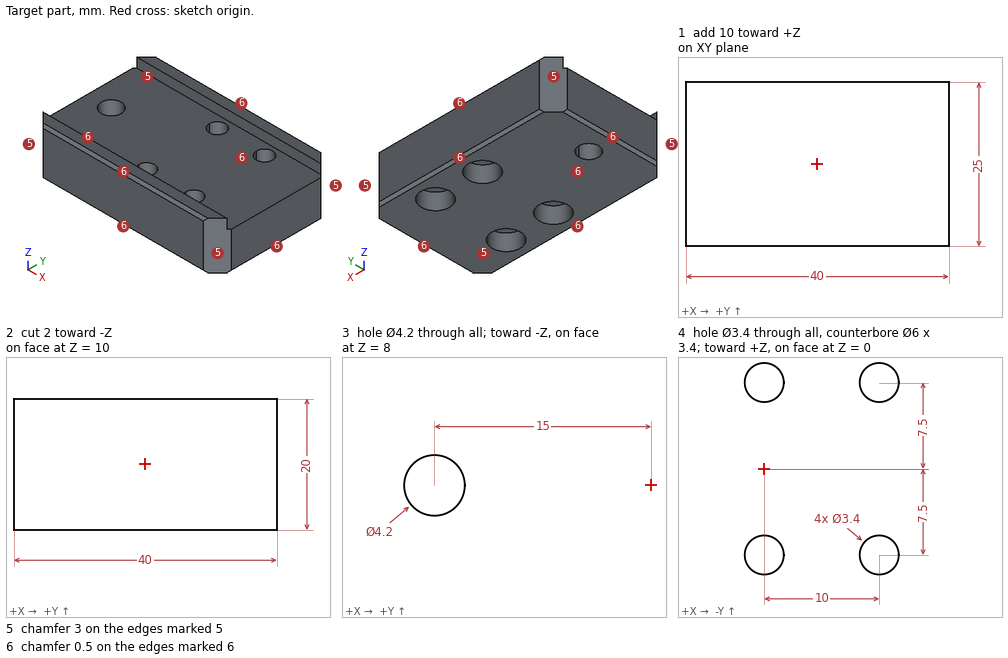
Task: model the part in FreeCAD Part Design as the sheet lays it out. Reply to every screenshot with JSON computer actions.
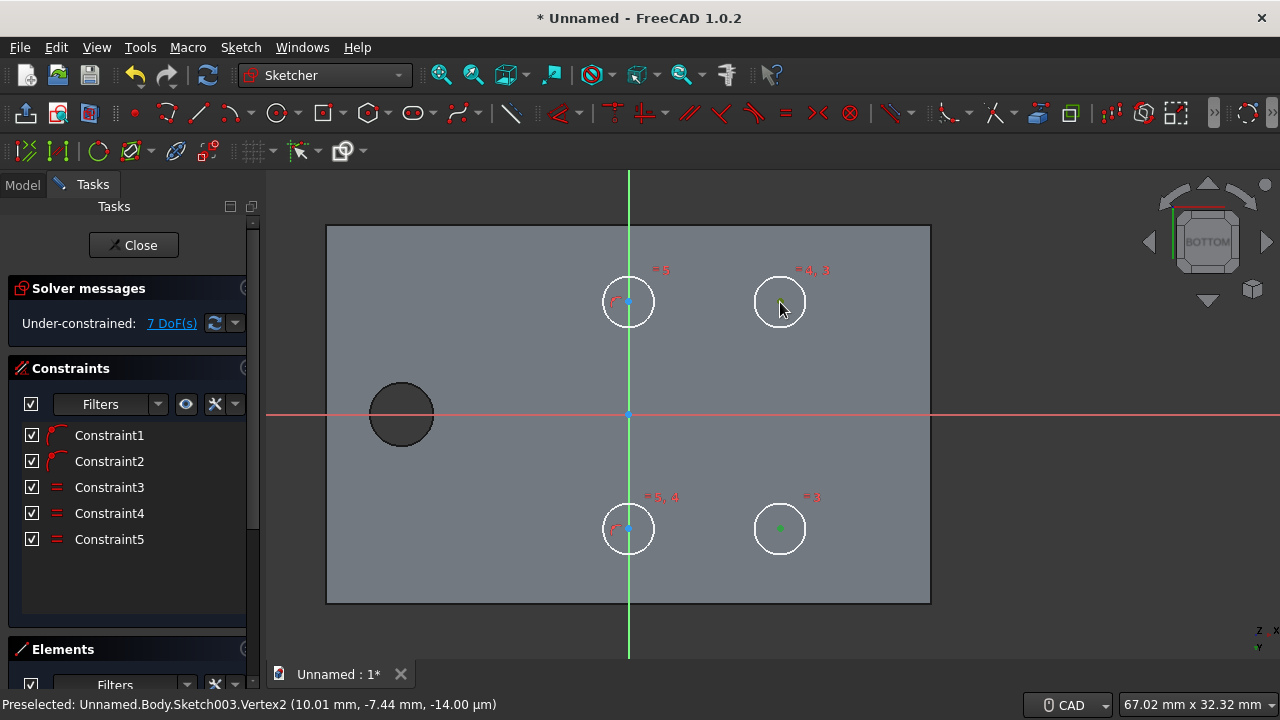
{"action": "key", "text": "v"}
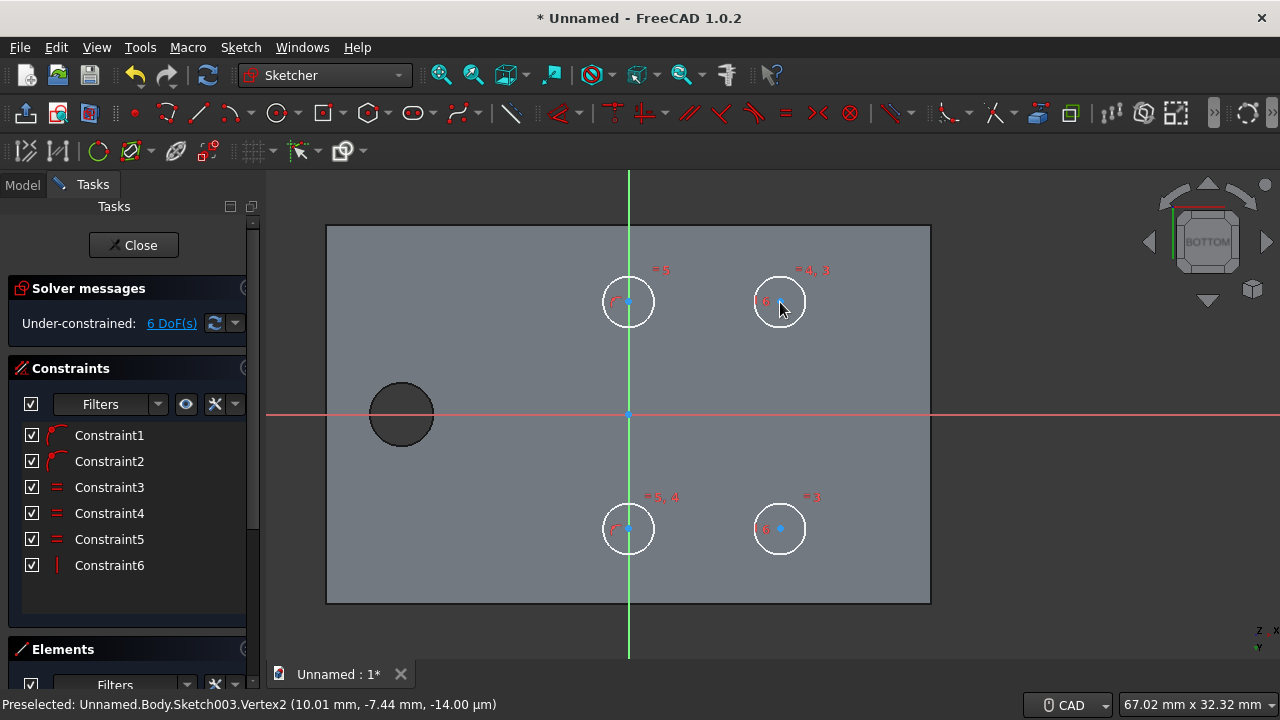
{"action": "left_click", "coordinate": [780, 529]}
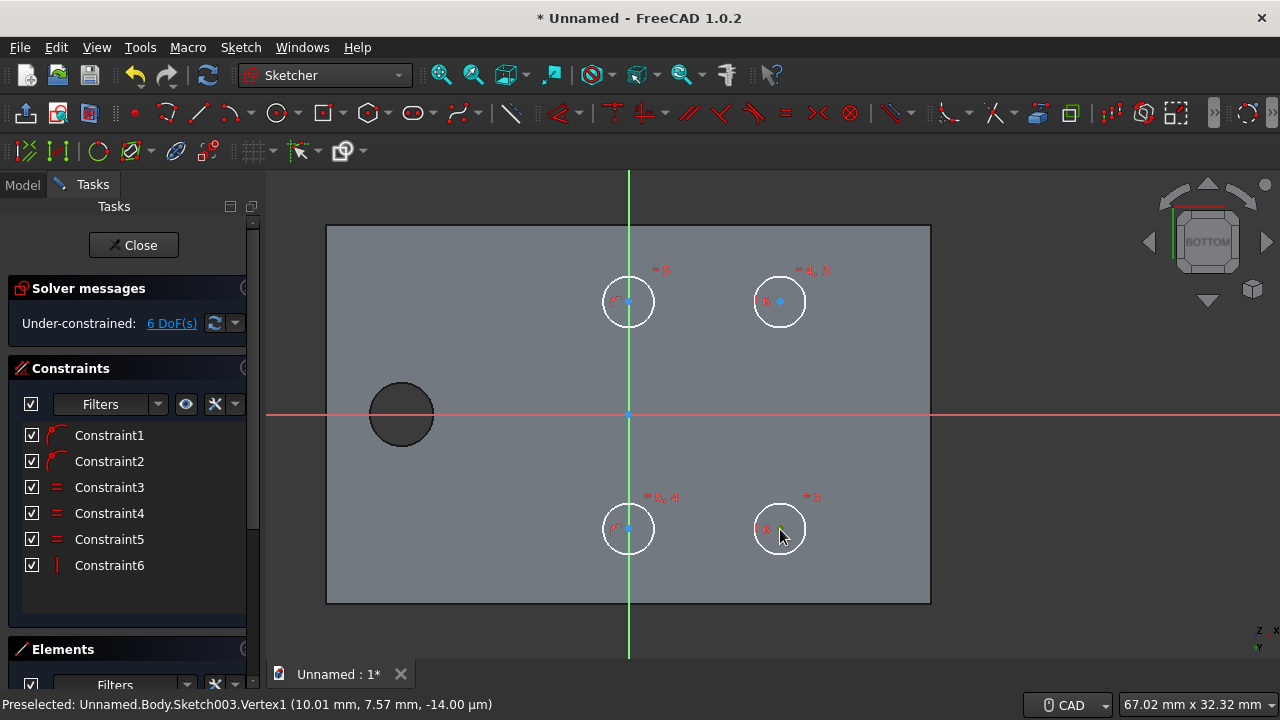
{"action": "left_click", "coordinate": [629, 529]}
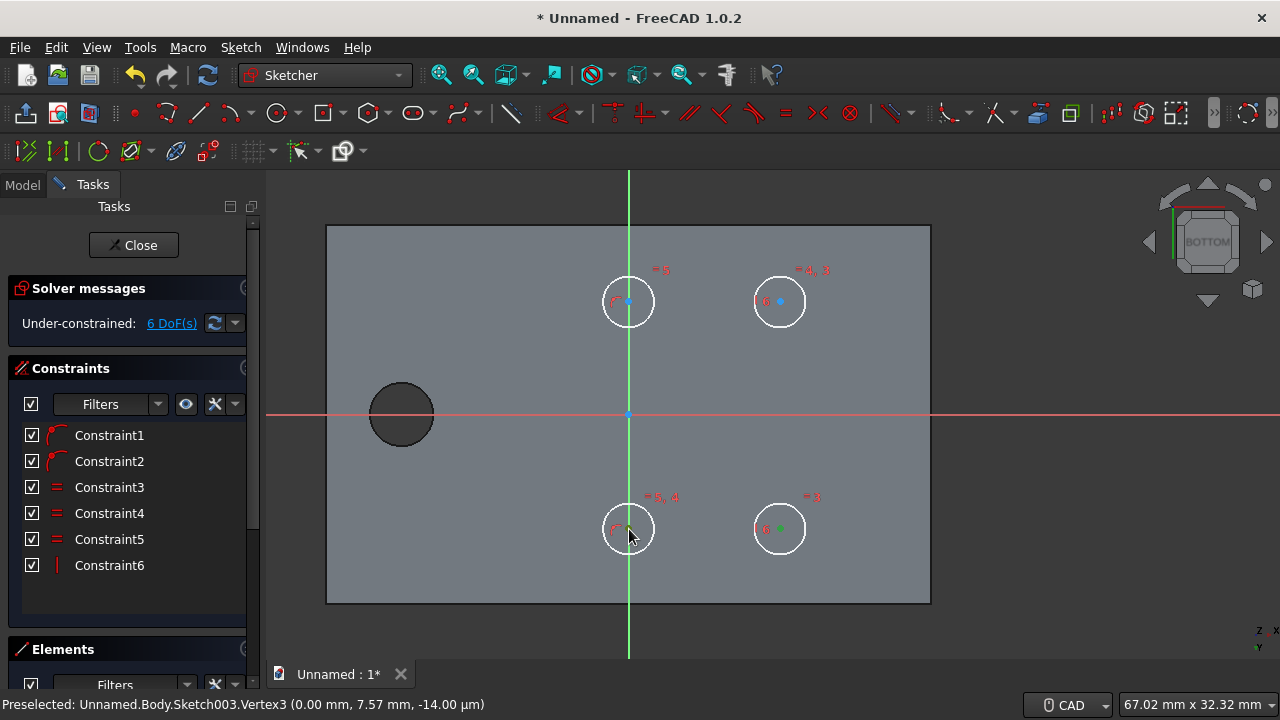
{"action": "key", "text": "h"}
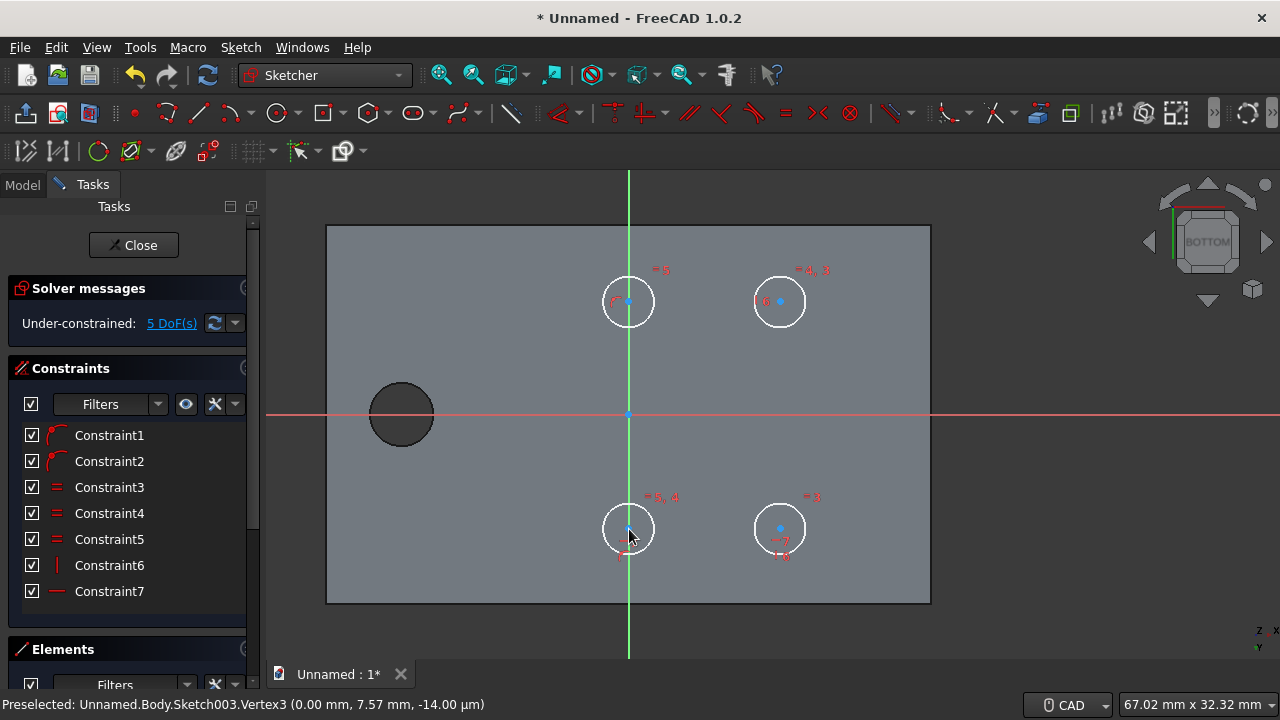
{"action": "left_click", "coordinate": [780, 302]}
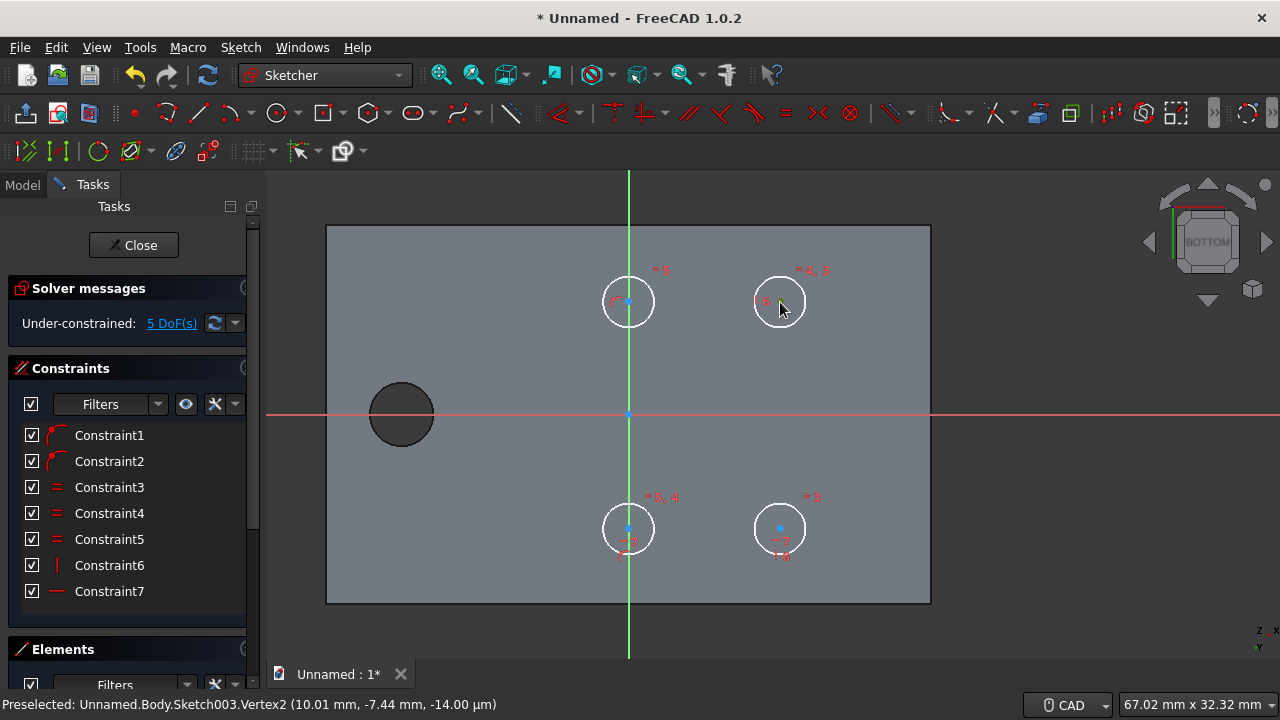
{"action": "left_click", "coordinate": [629, 302]}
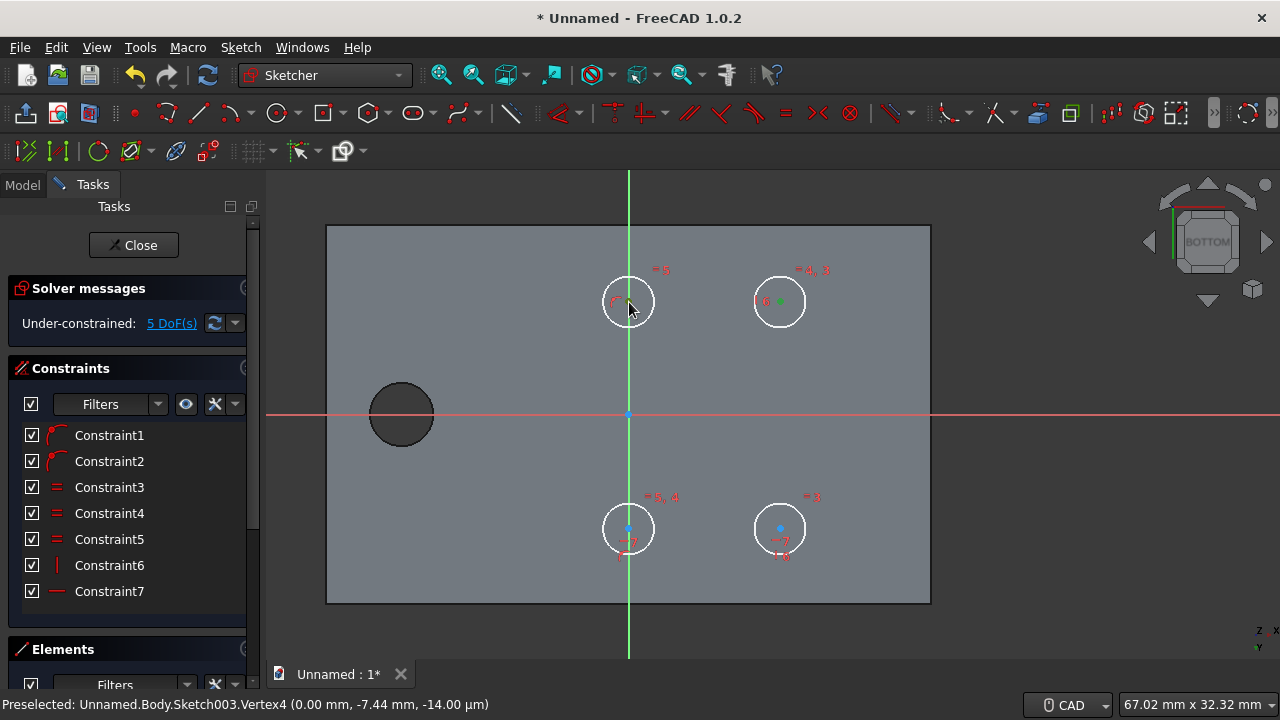
{"action": "left_click", "coordinate": [668, 114]}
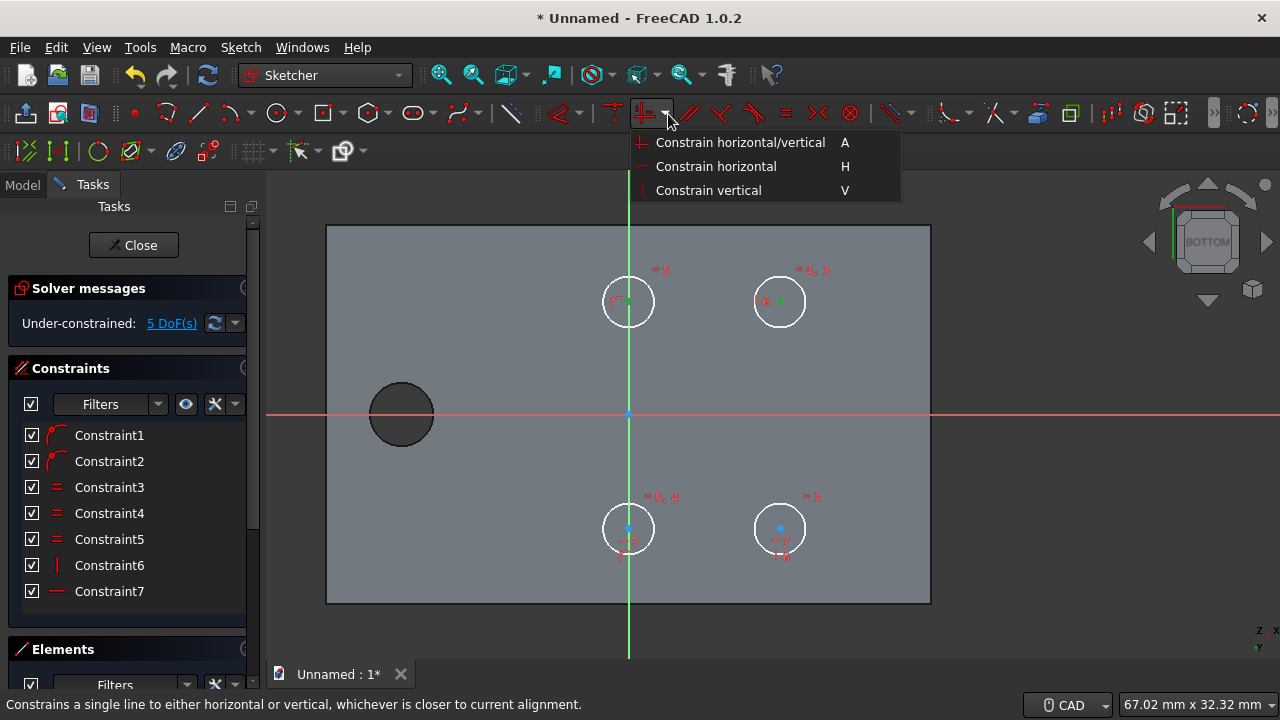
{"action": "left_click", "coordinate": [766, 166]}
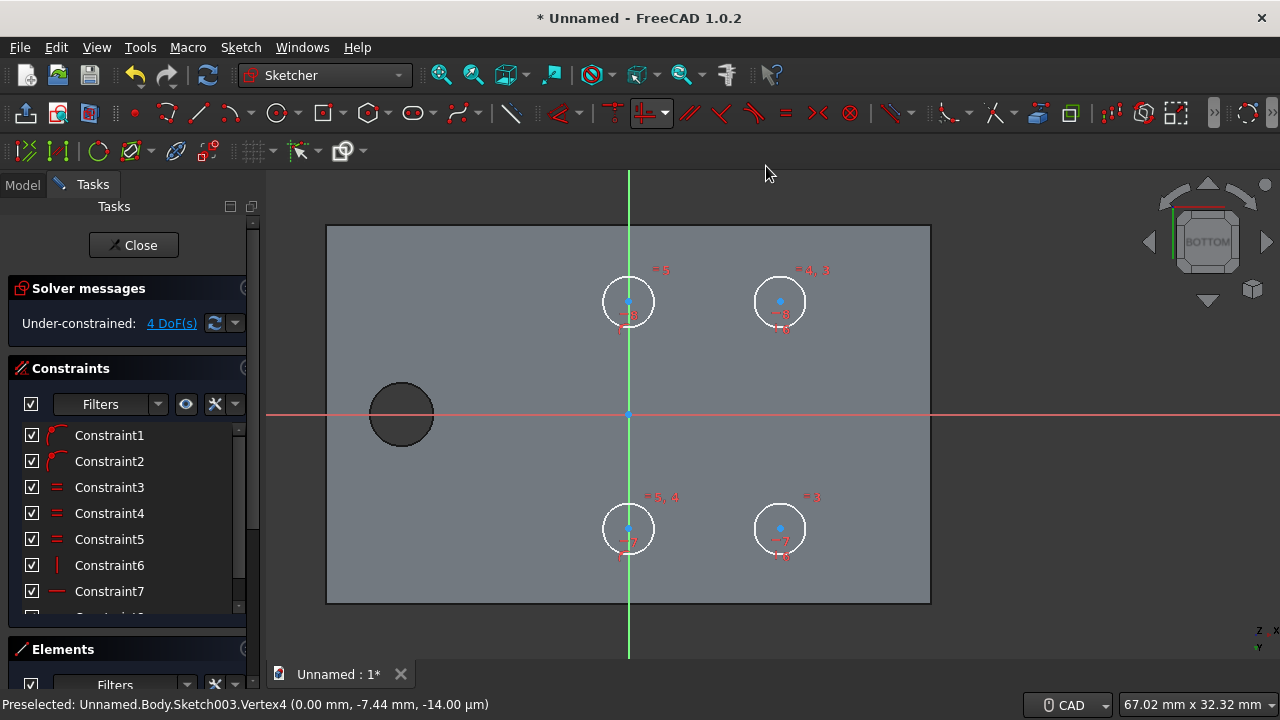
{"action": "left_click", "coordinate": [558, 114]}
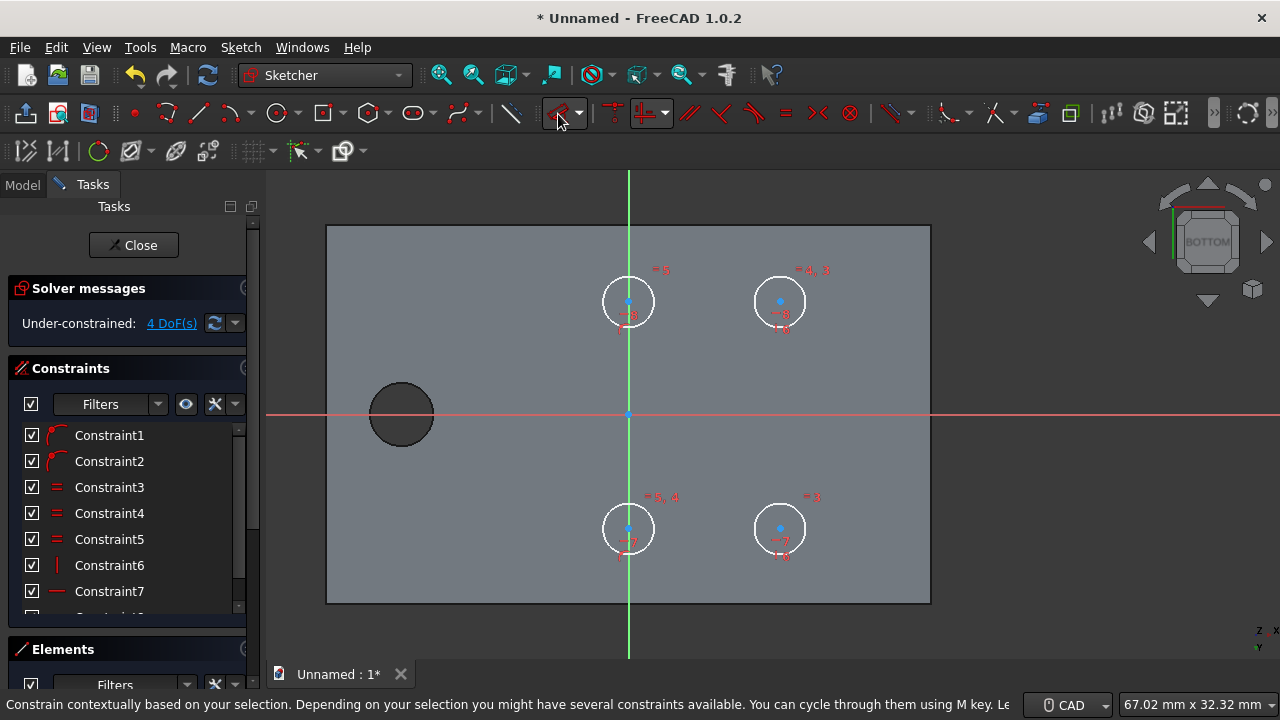
{"action": "left_click", "coordinate": [798, 511]}
{"action": "left_click", "coordinate": [821, 488]}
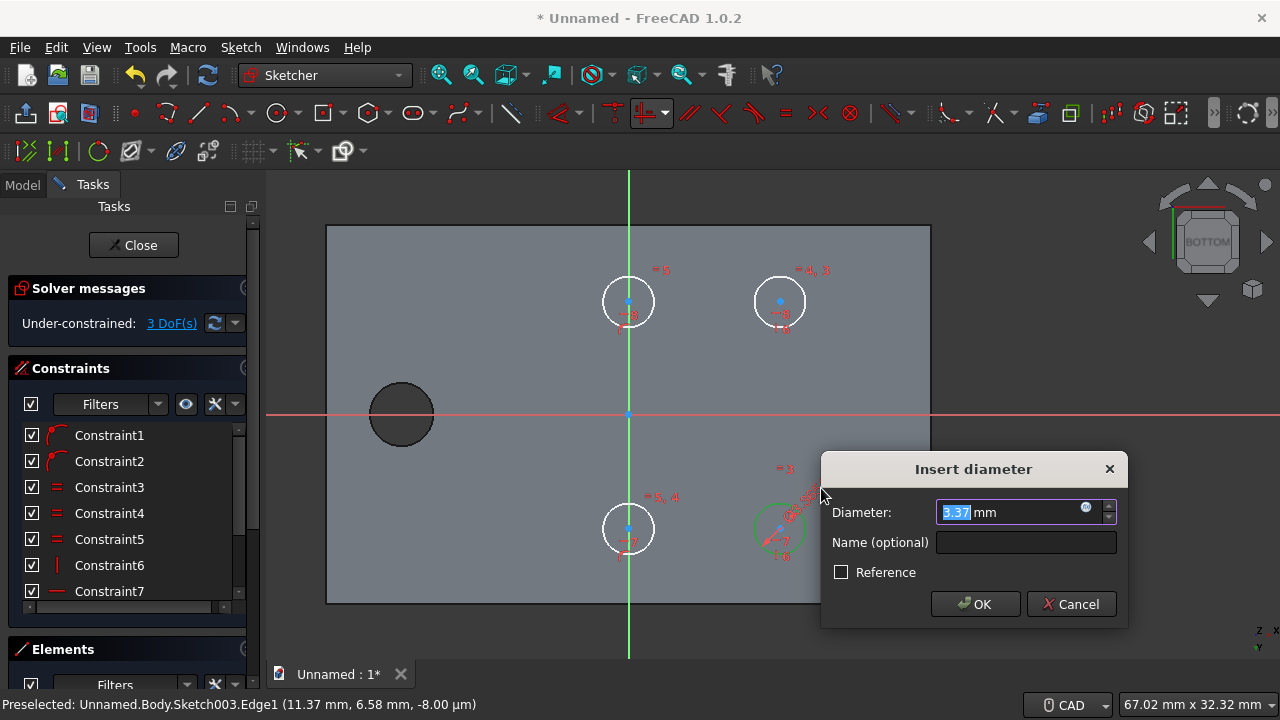
{"action": "type", "text": "3.4"}
{"action": "key", "text": "Return"}